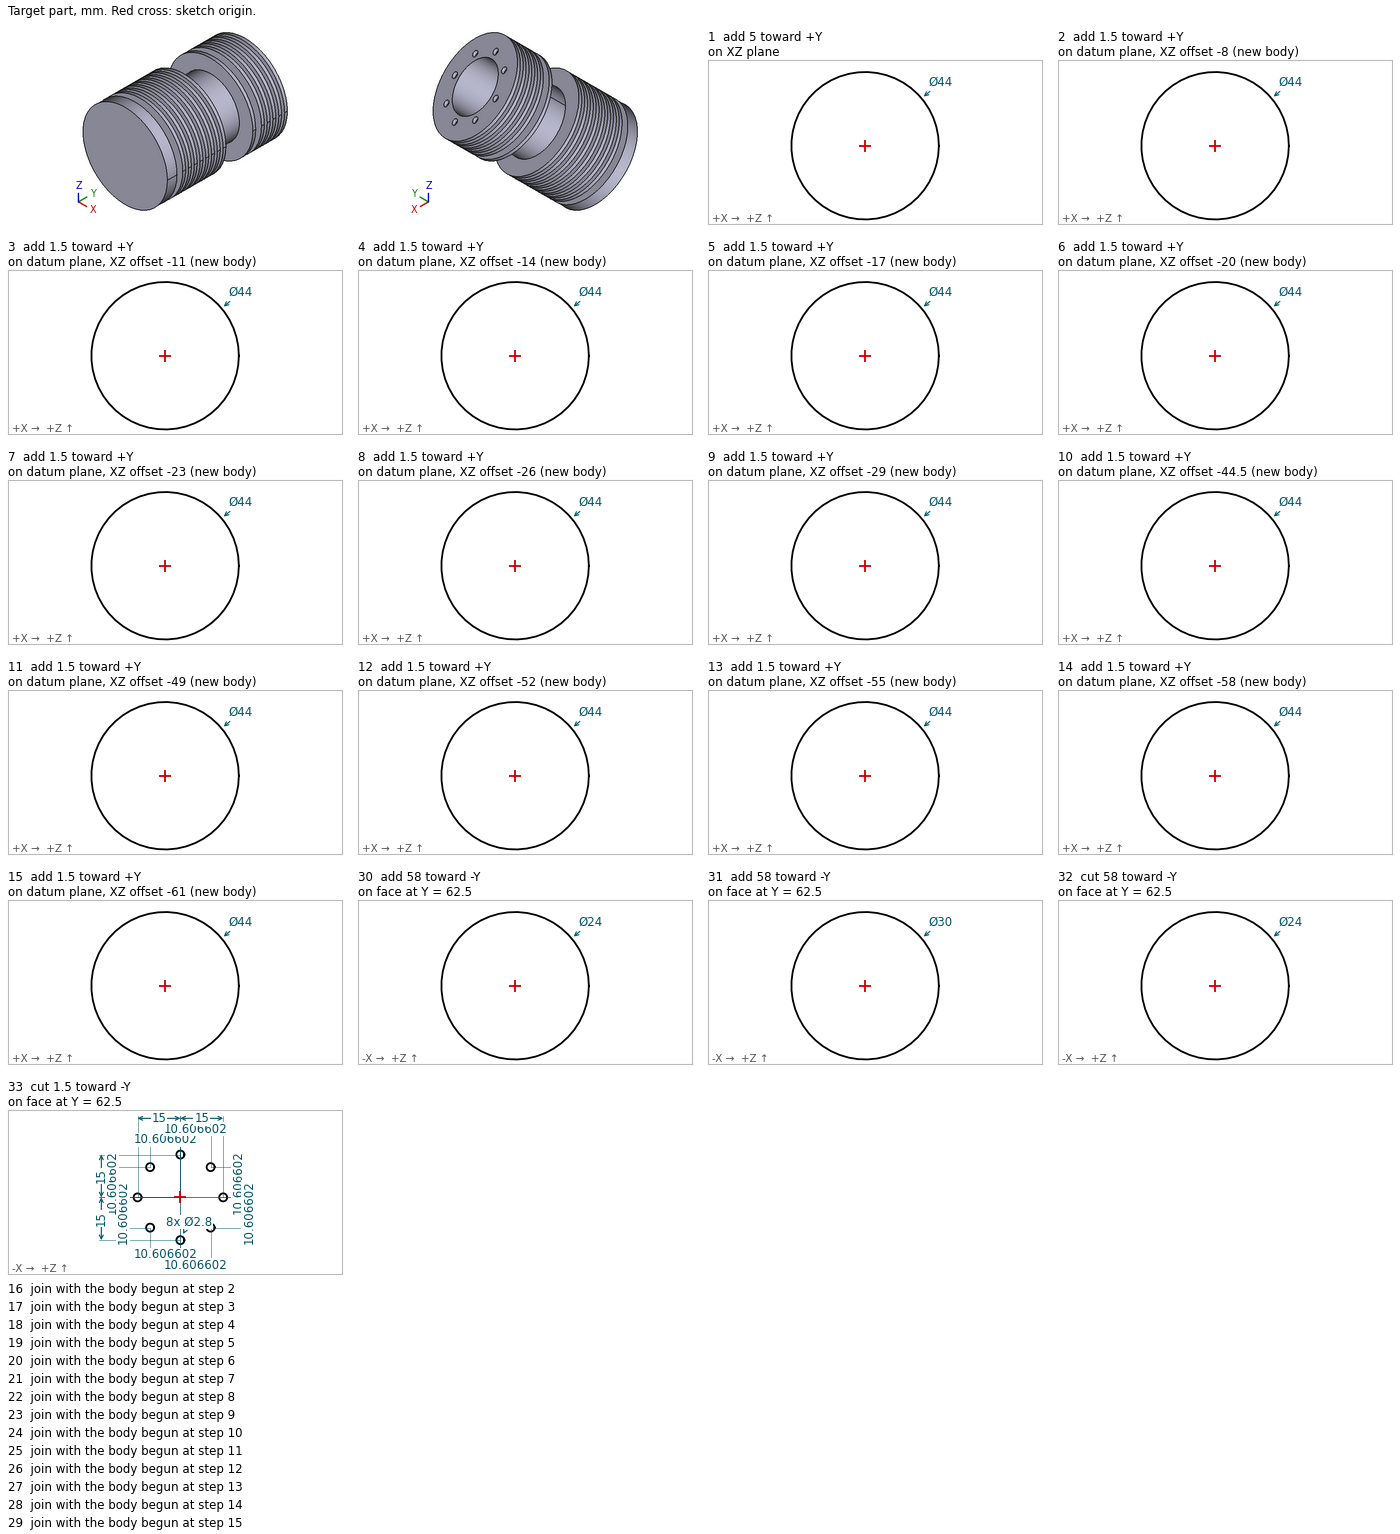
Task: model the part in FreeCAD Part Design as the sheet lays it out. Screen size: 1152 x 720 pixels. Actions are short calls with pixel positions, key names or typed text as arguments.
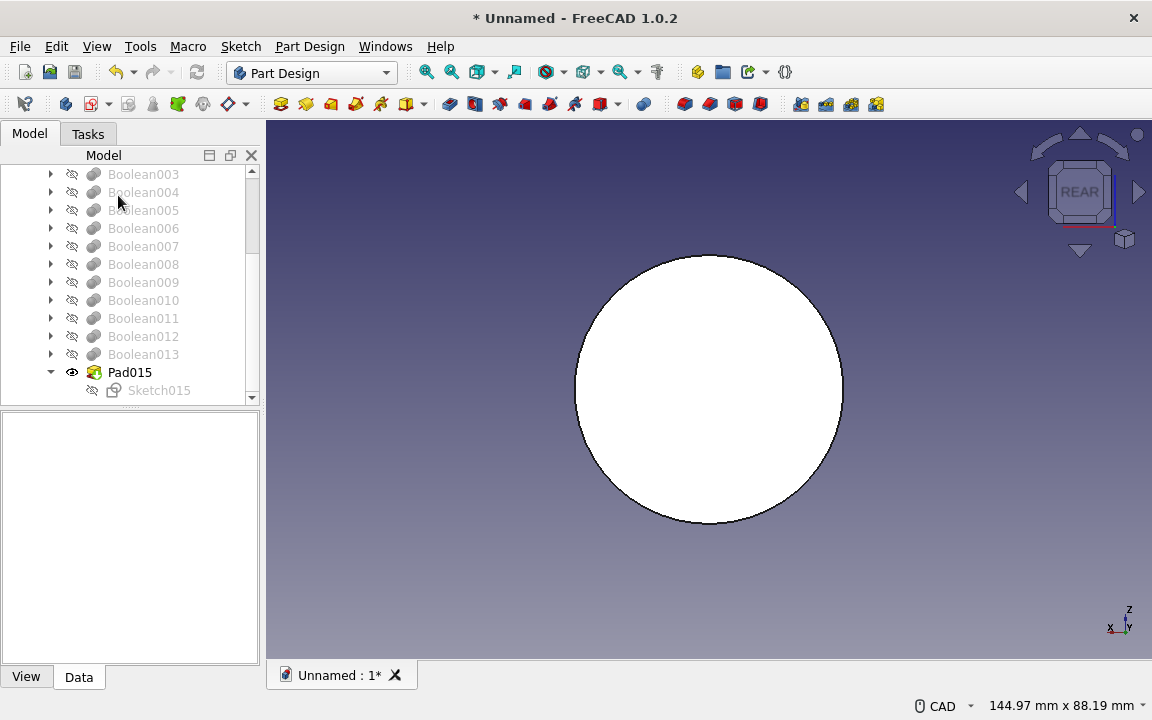
click(709, 389)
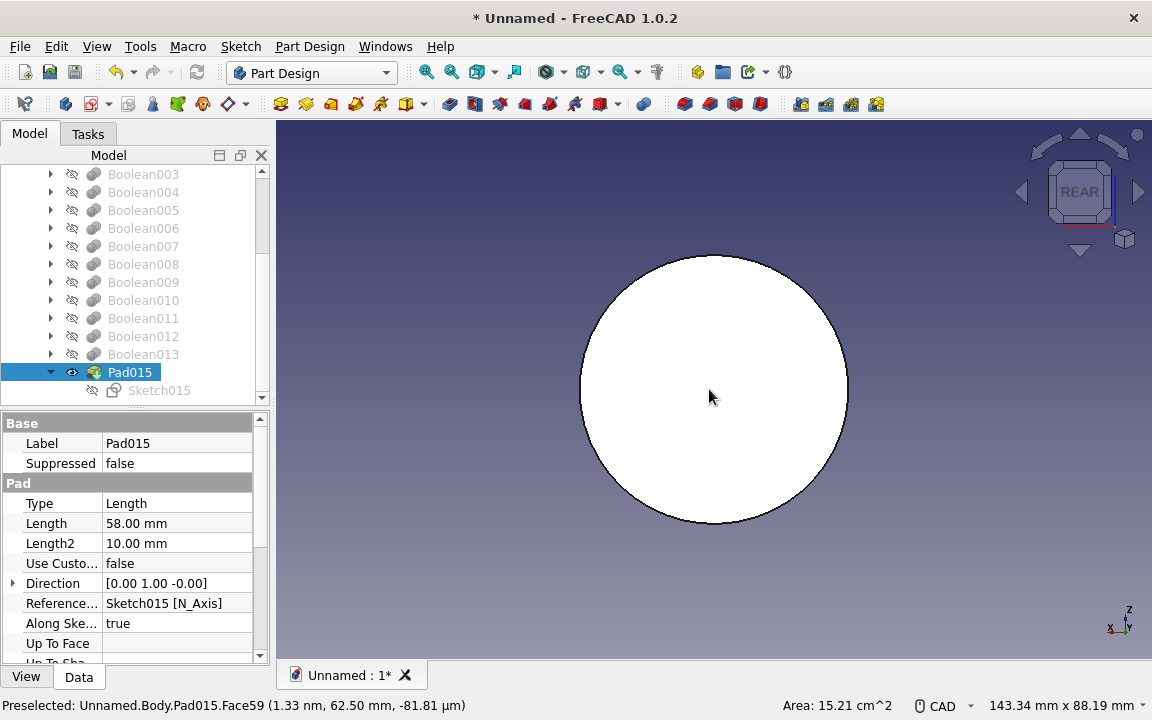
click(90, 104)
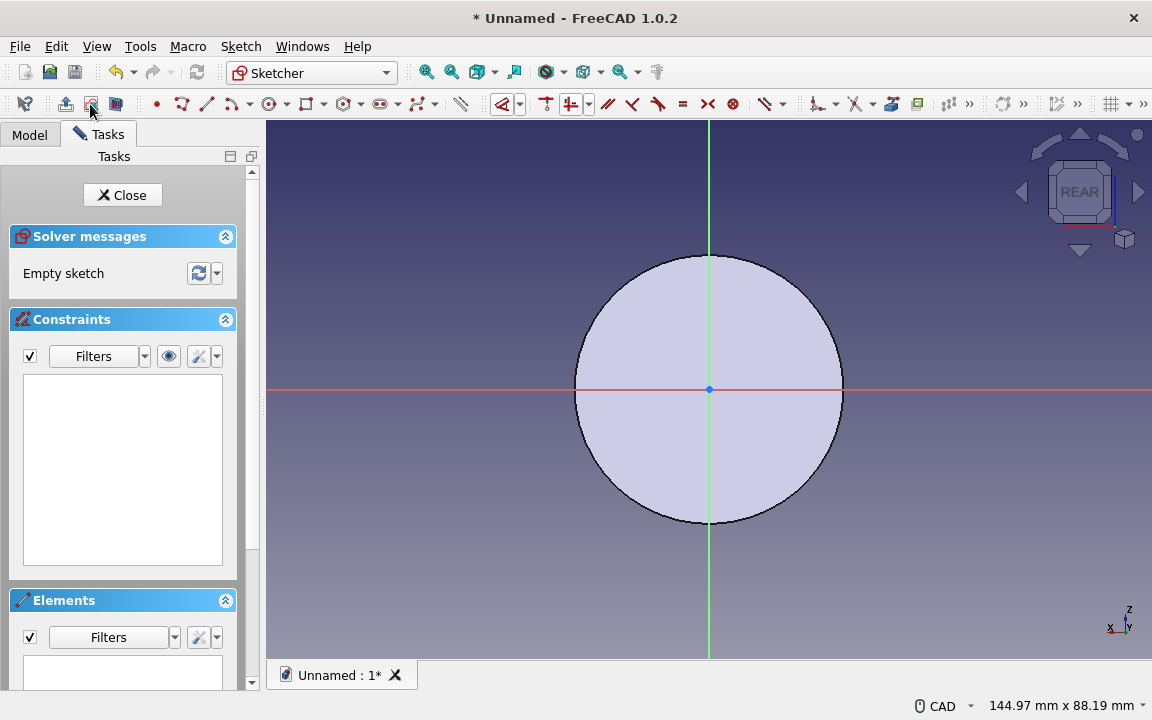
scroll(792, 390, up, 3)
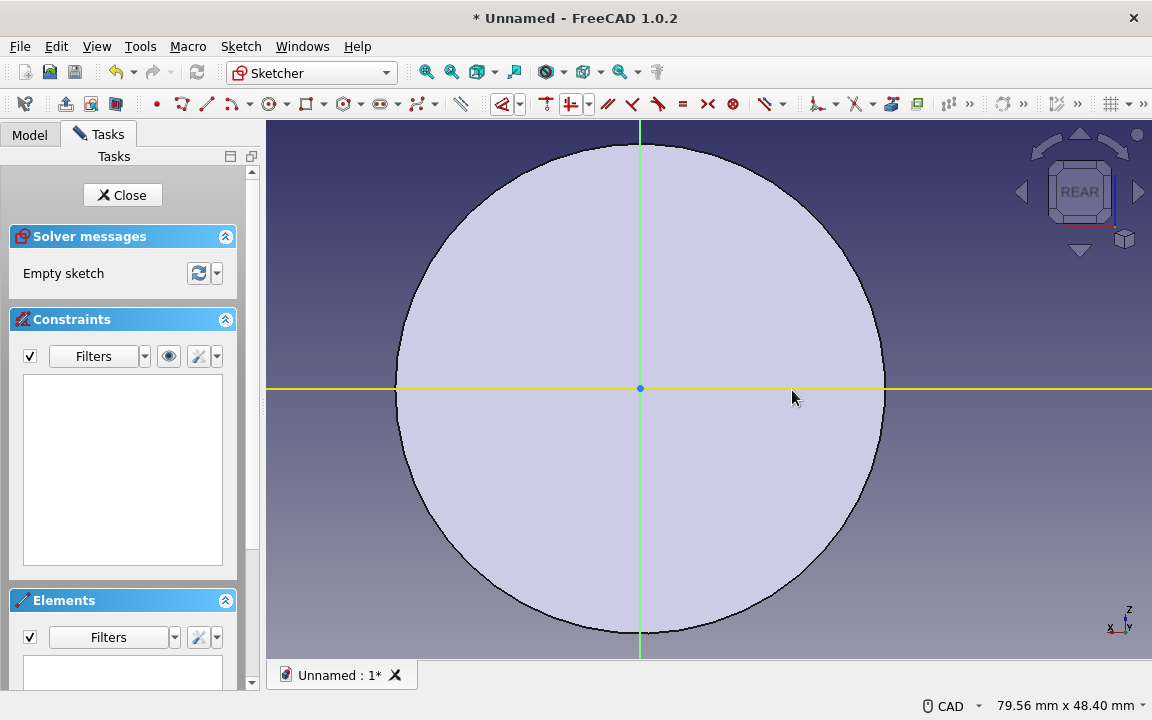
click(268, 104)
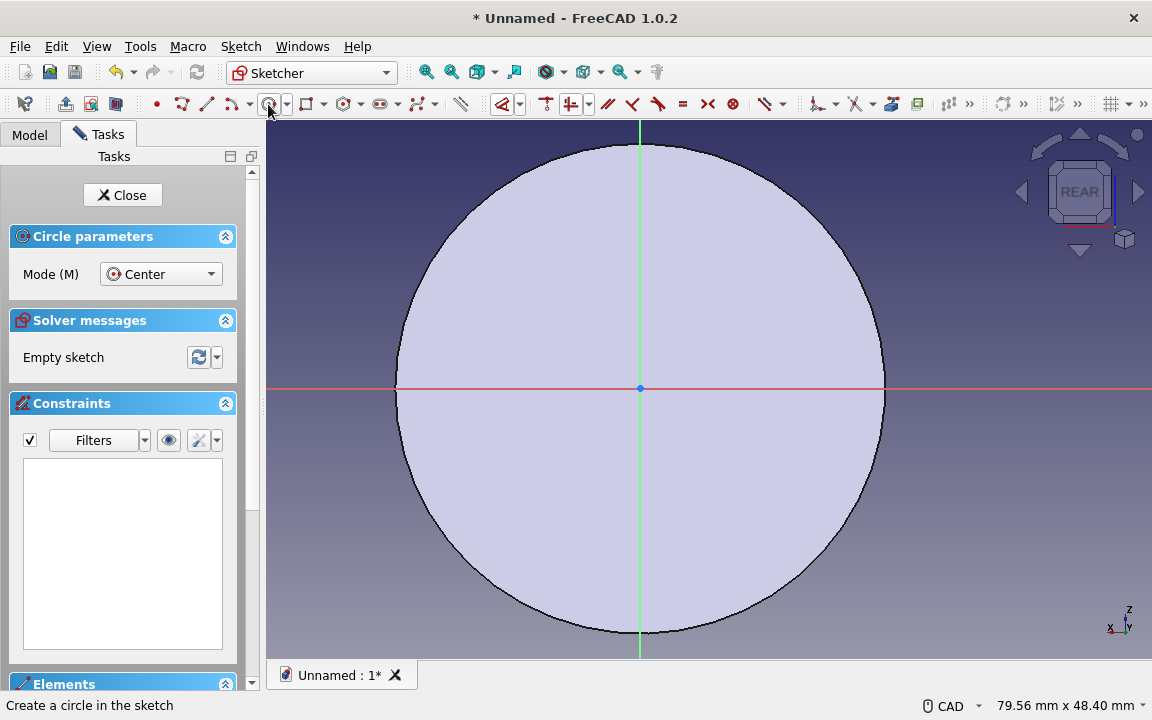
click(640, 389)
click(758, 271)
key(Escape)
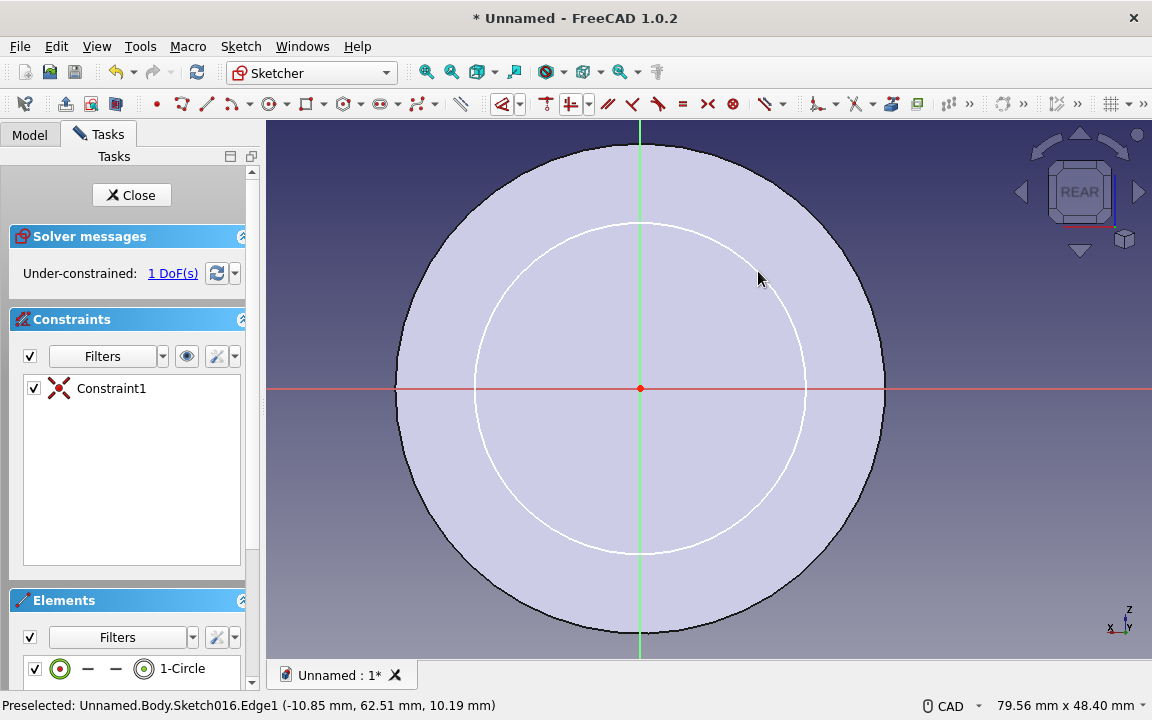
click(757, 271)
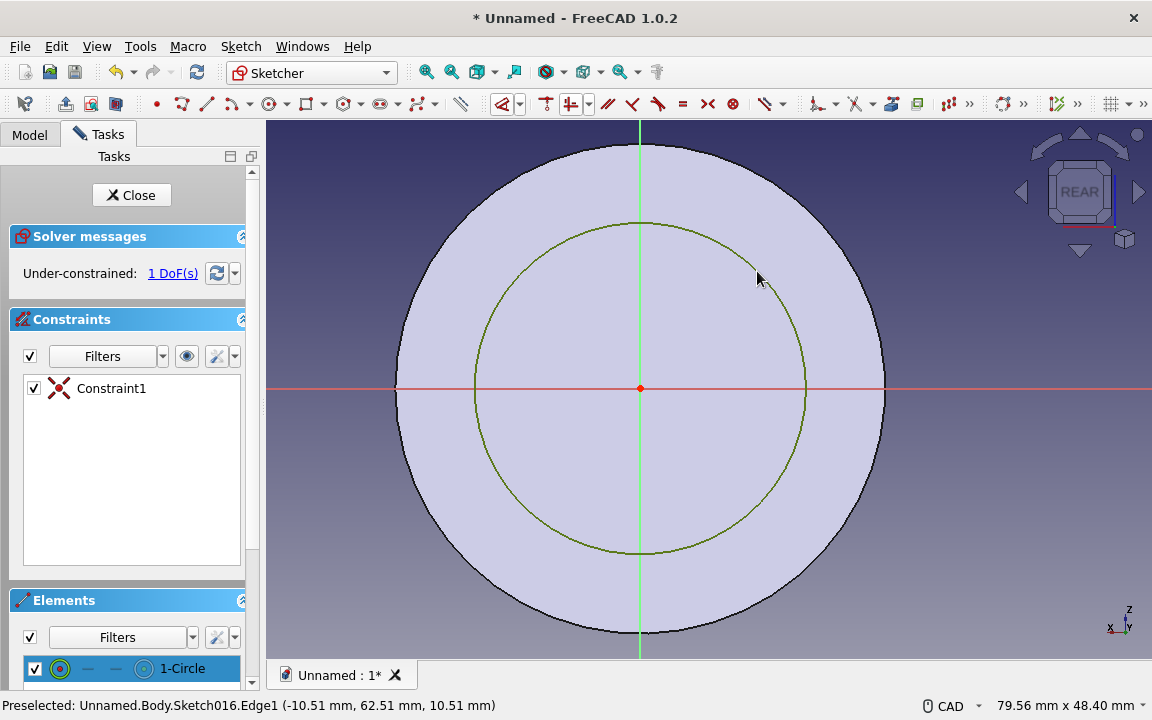
key(k)
key(o)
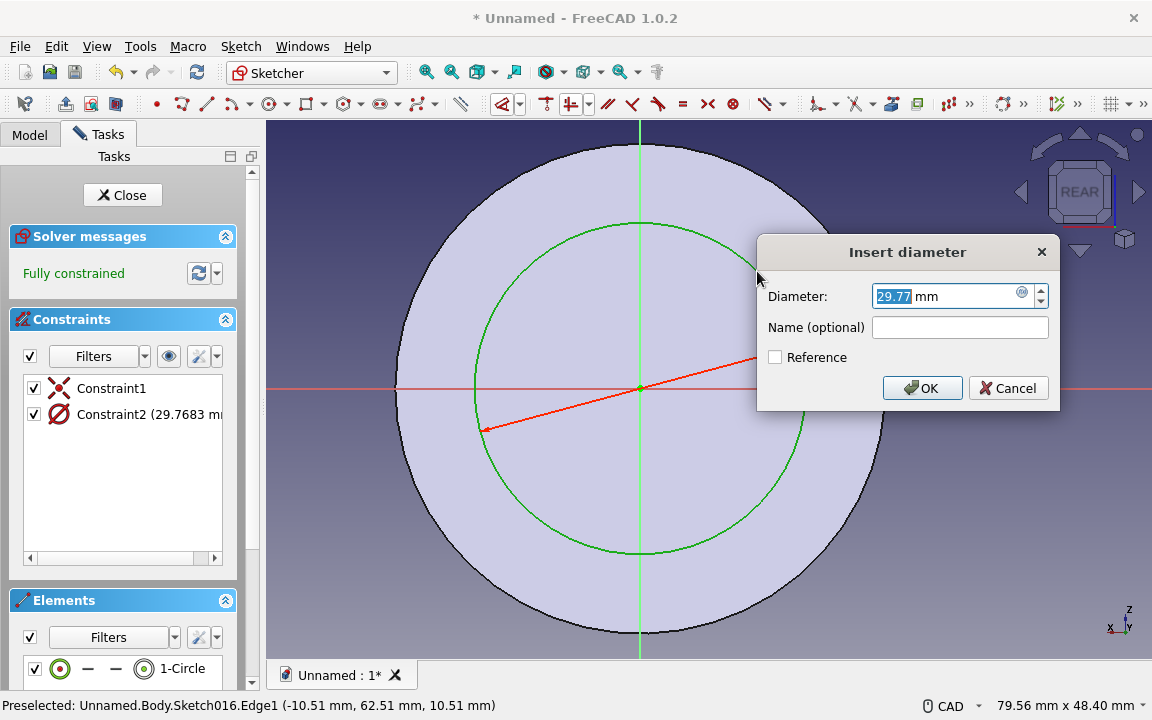
text(30)
key(Return)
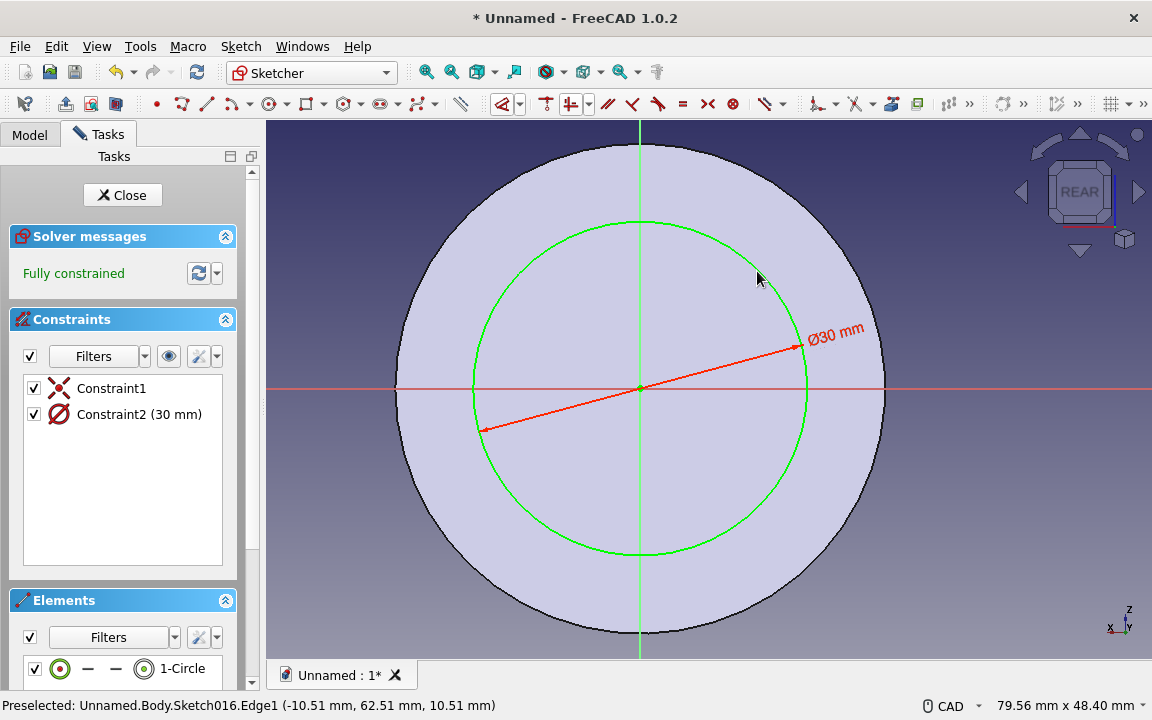
click(123, 195)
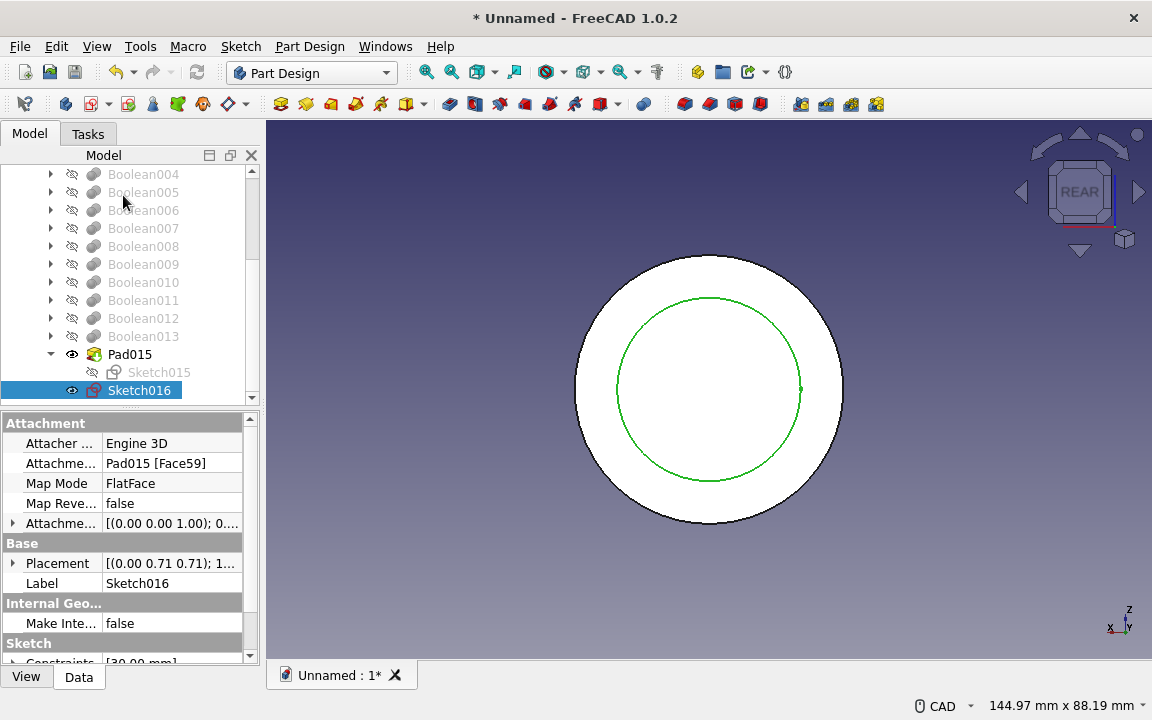
click(281, 104)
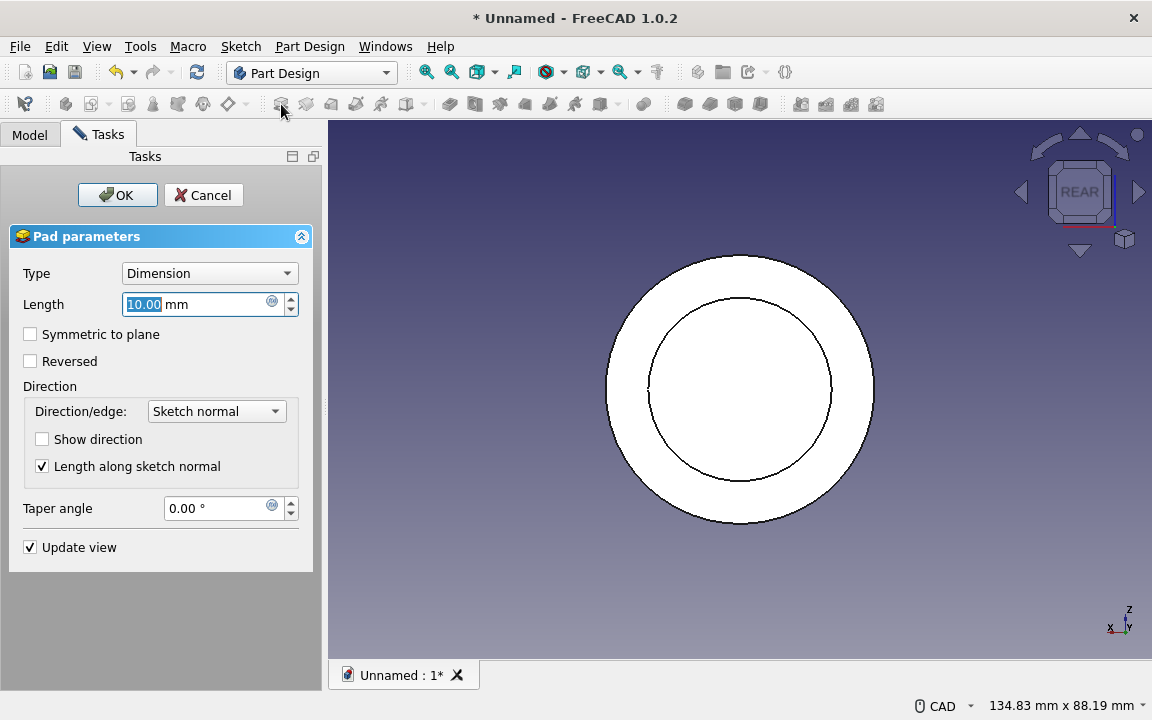
text(58)
key(Tab)